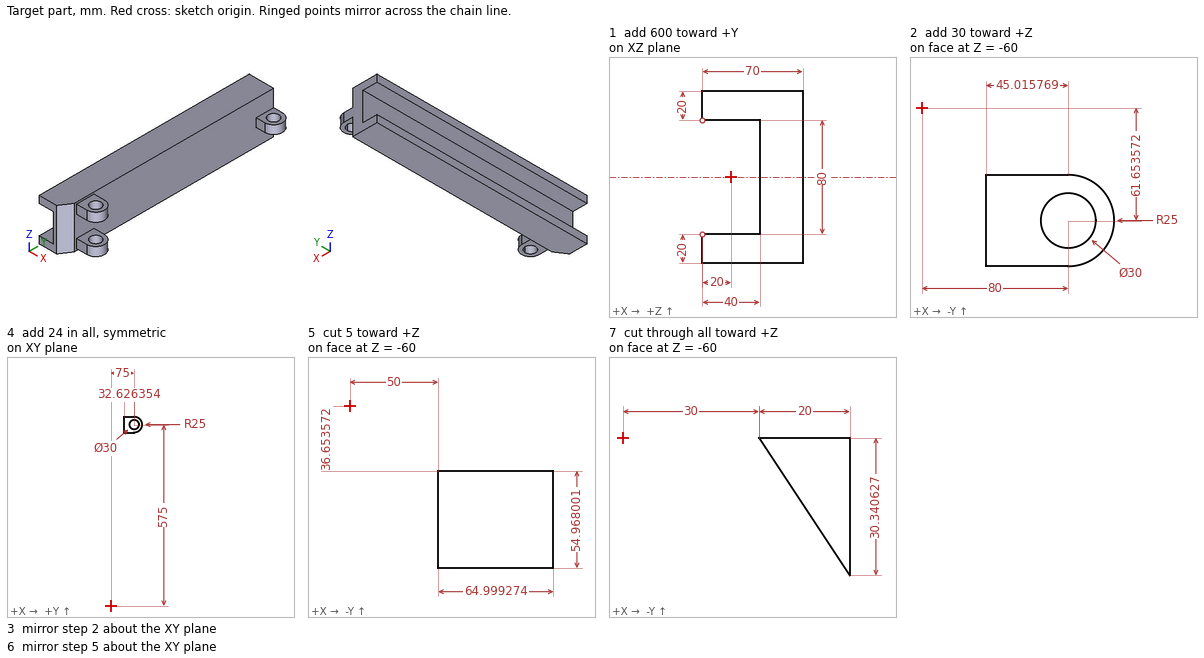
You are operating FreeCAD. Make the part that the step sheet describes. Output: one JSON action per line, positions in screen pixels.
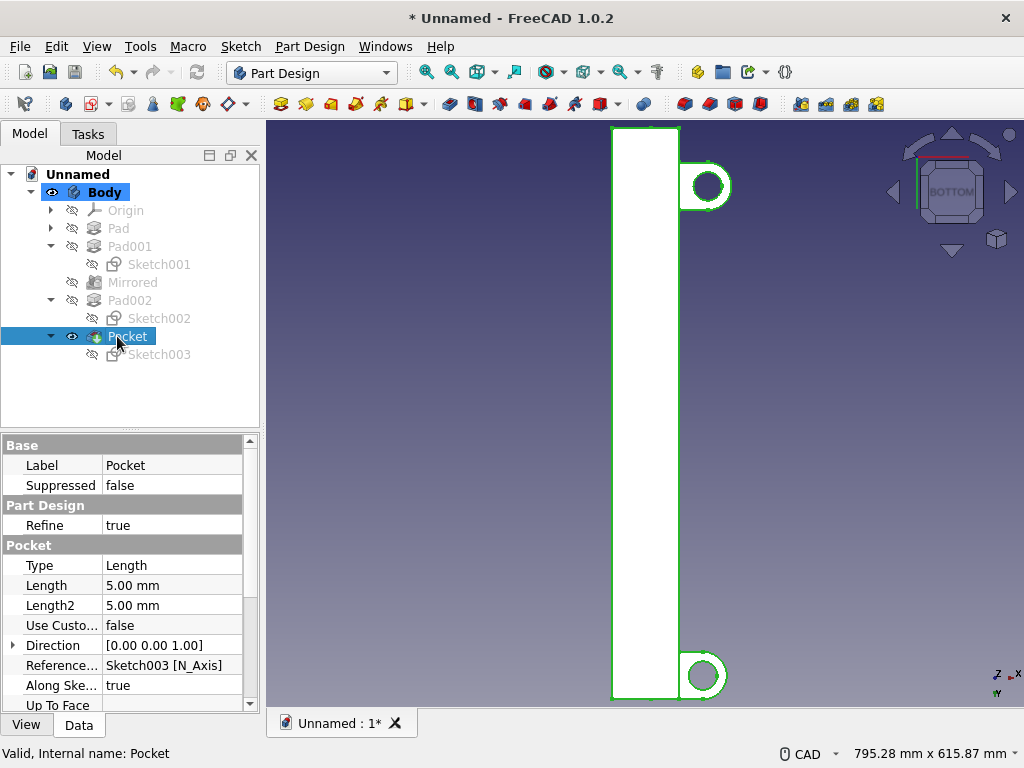
{"action": "left_click", "coordinate": [801, 104]}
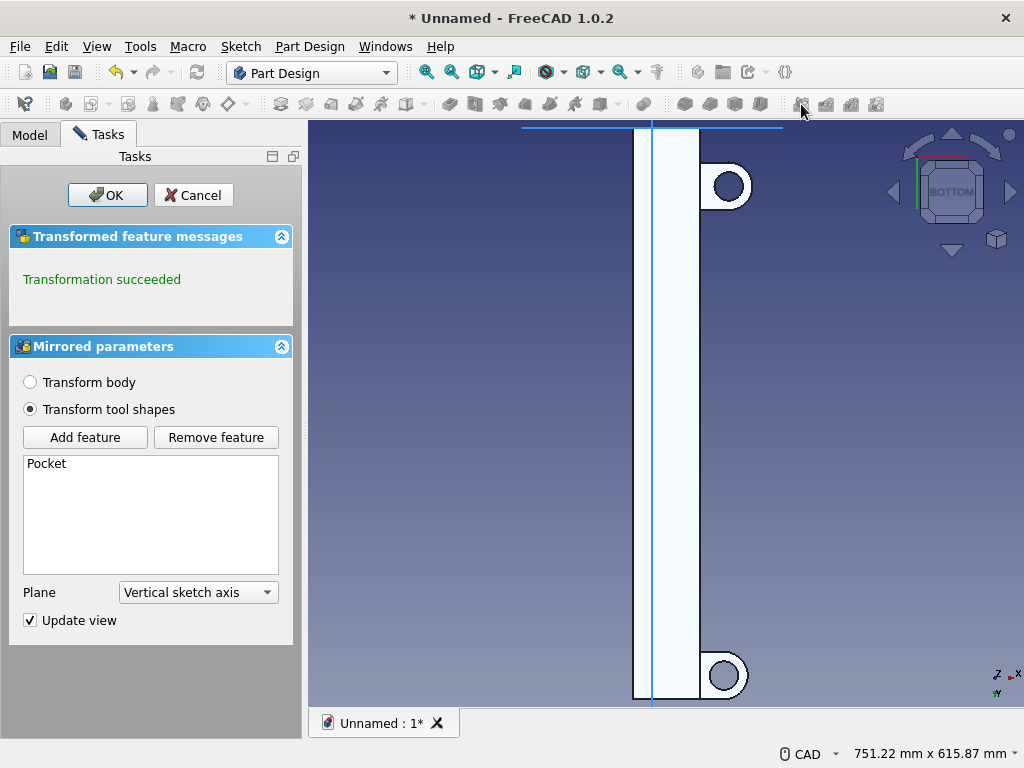
{"action": "left_click", "coordinate": [199, 592]}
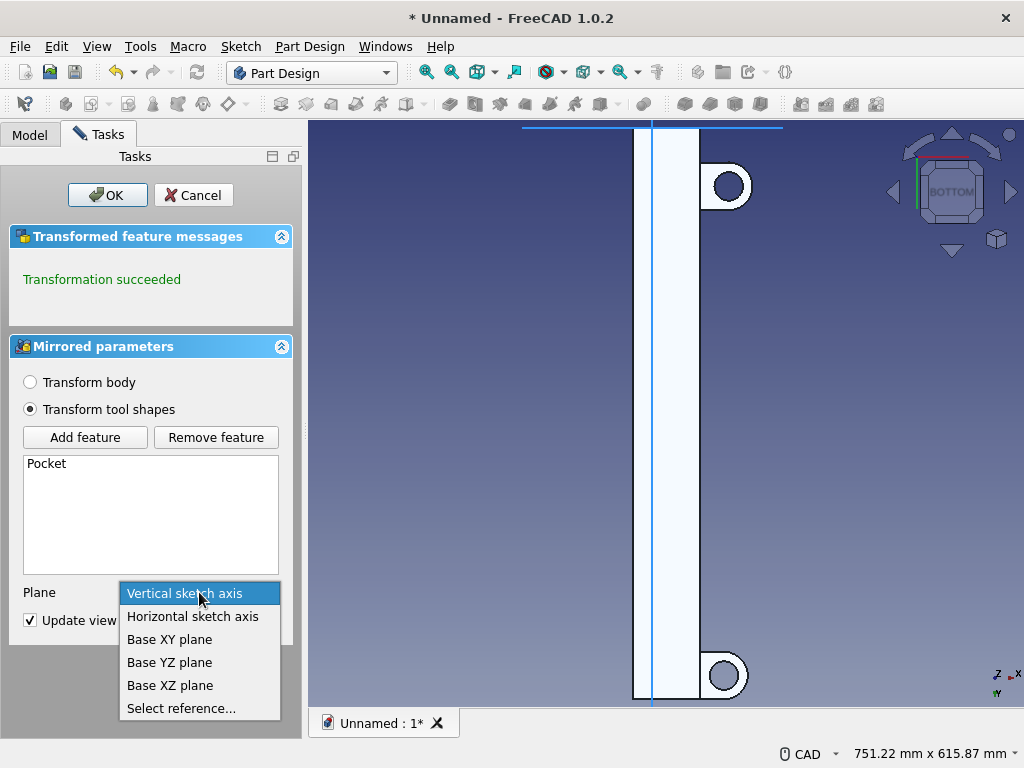
{"action": "left_click", "coordinate": [198, 640]}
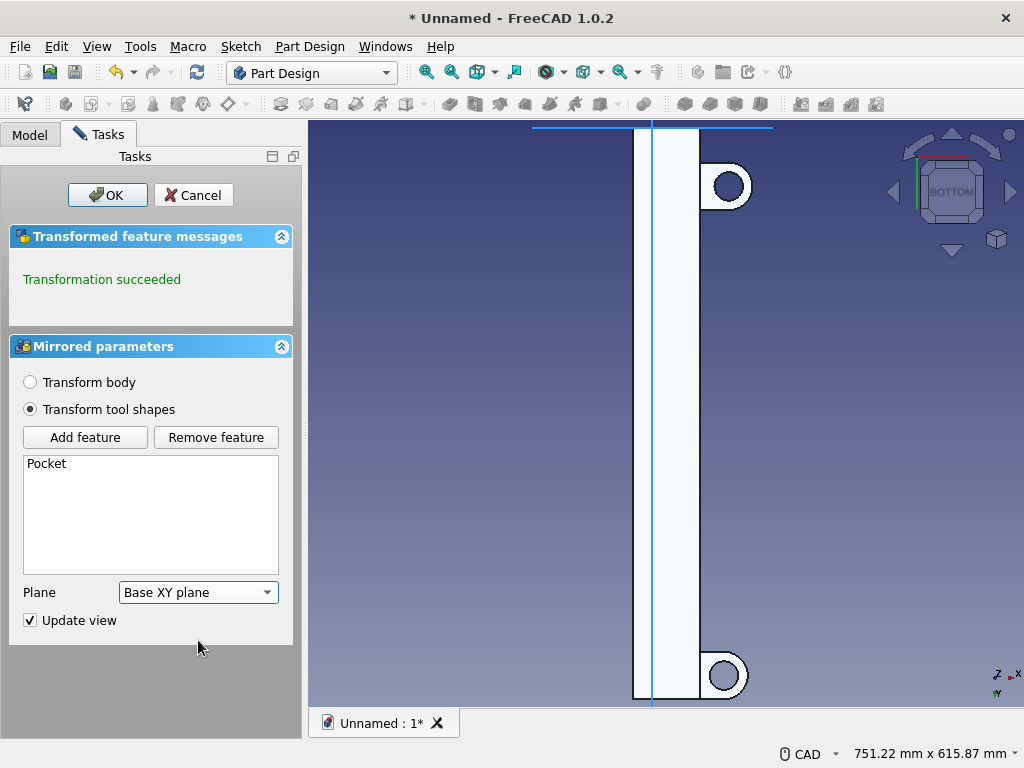
{"action": "left_click", "coordinate": [108, 195]}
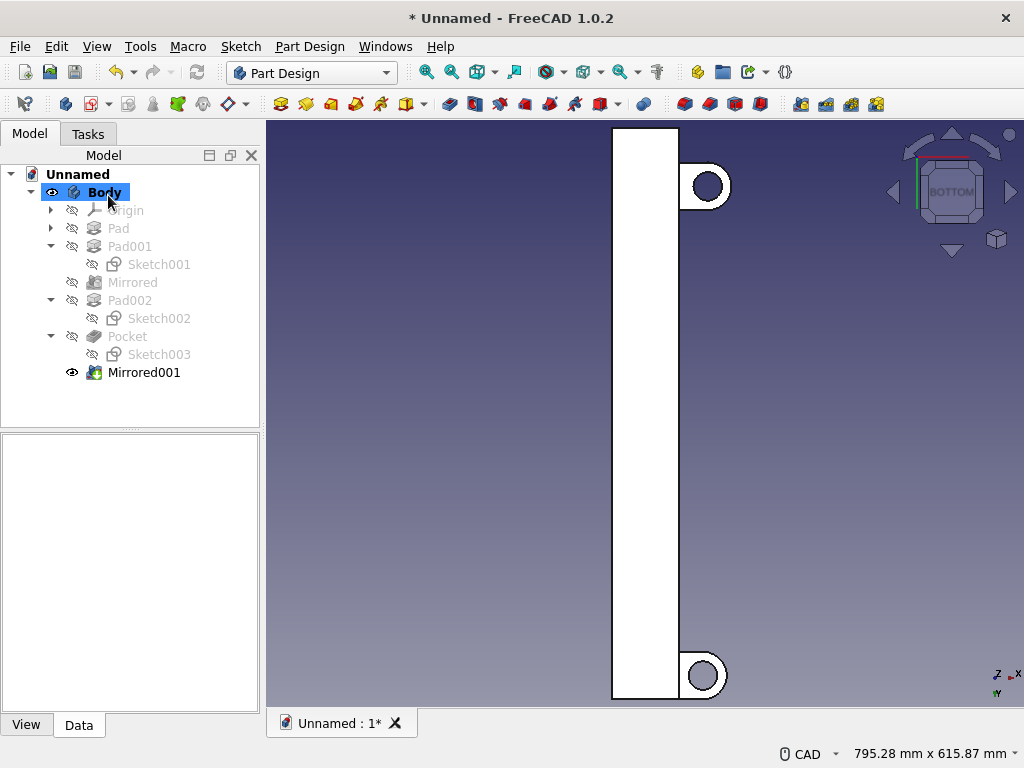
{"action": "left_click", "coordinate": [646, 658]}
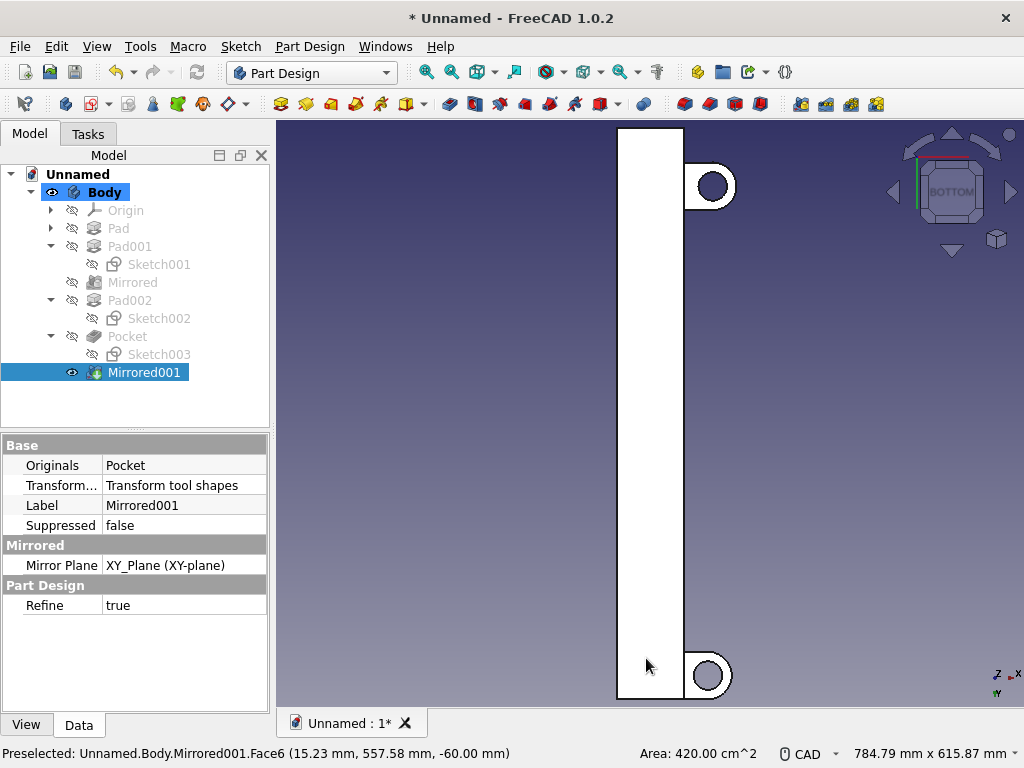
{"action": "left_click", "coordinate": [90, 104]}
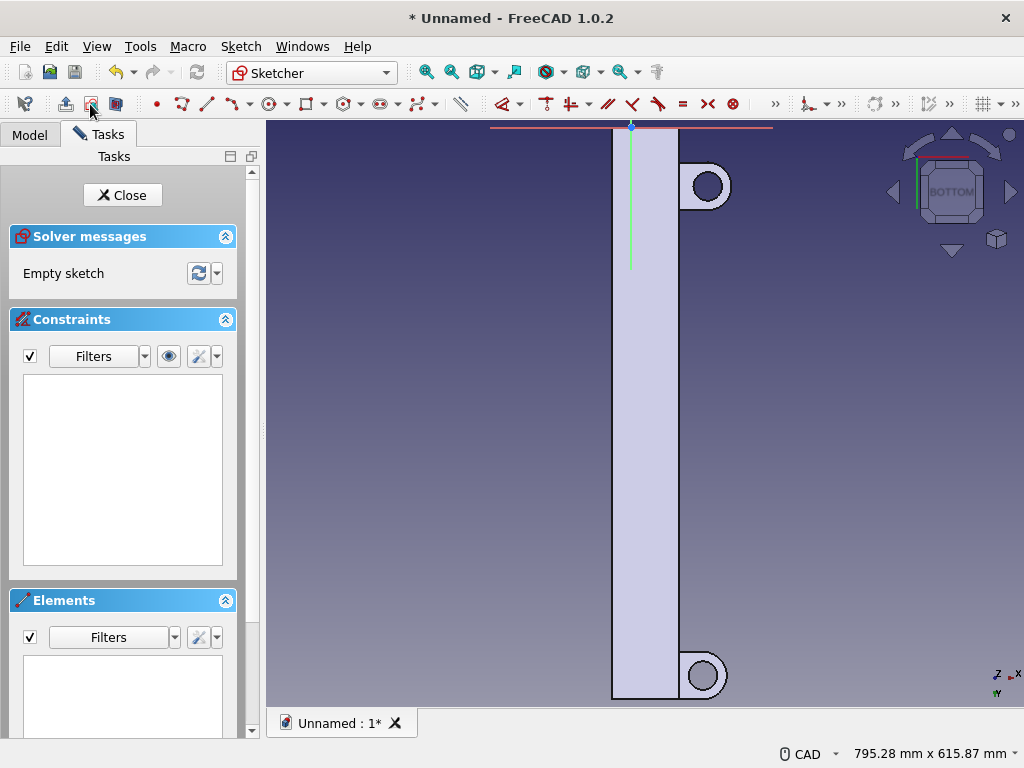
{"action": "scroll", "coordinate": [576, 414], "scroll_direction": "down", "scroll_amount": 5}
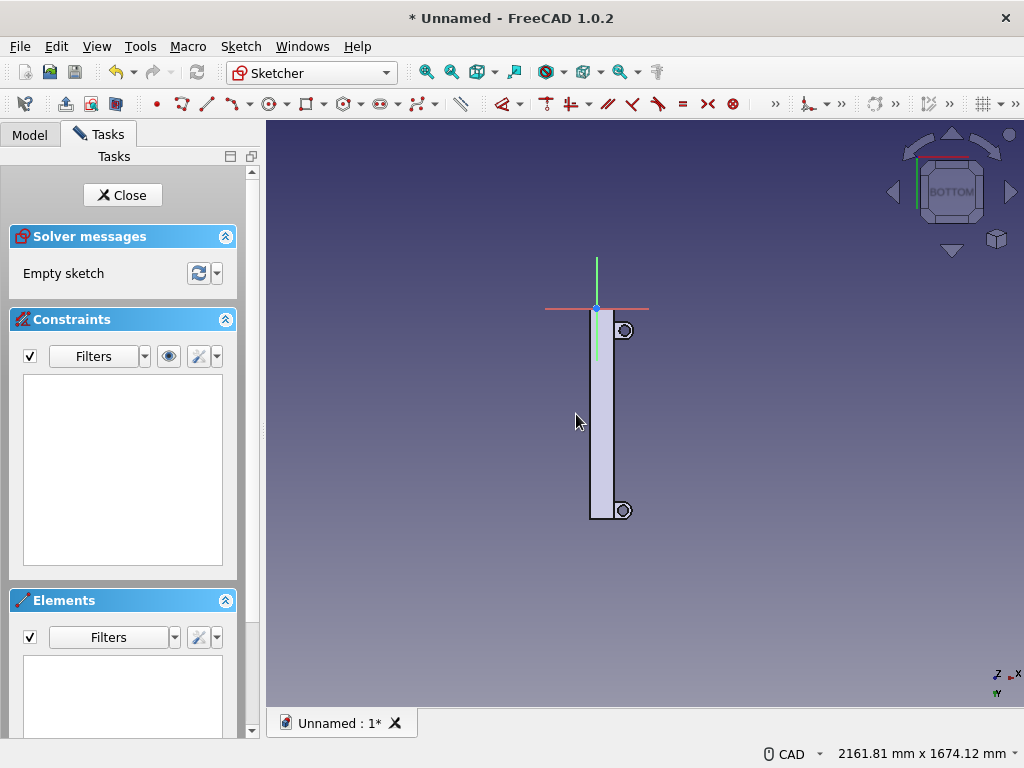
{"action": "scroll", "coordinate": [607, 309], "scroll_direction": "up", "scroll_amount": 15}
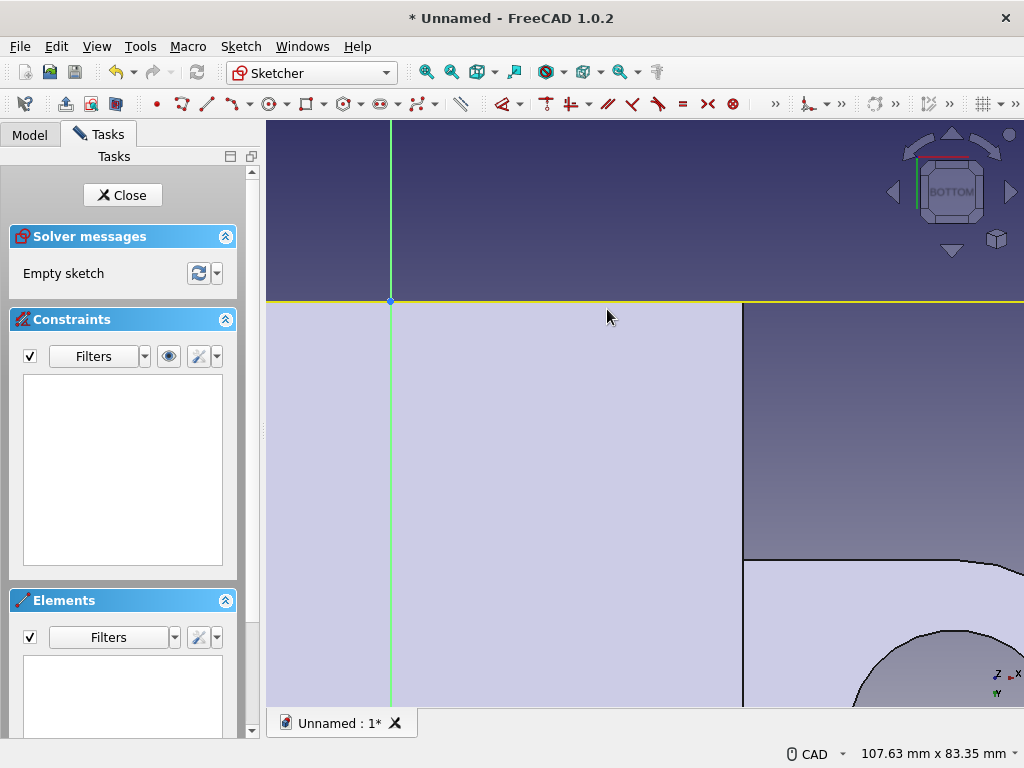
{"action": "left_click", "coordinate": [182, 104]}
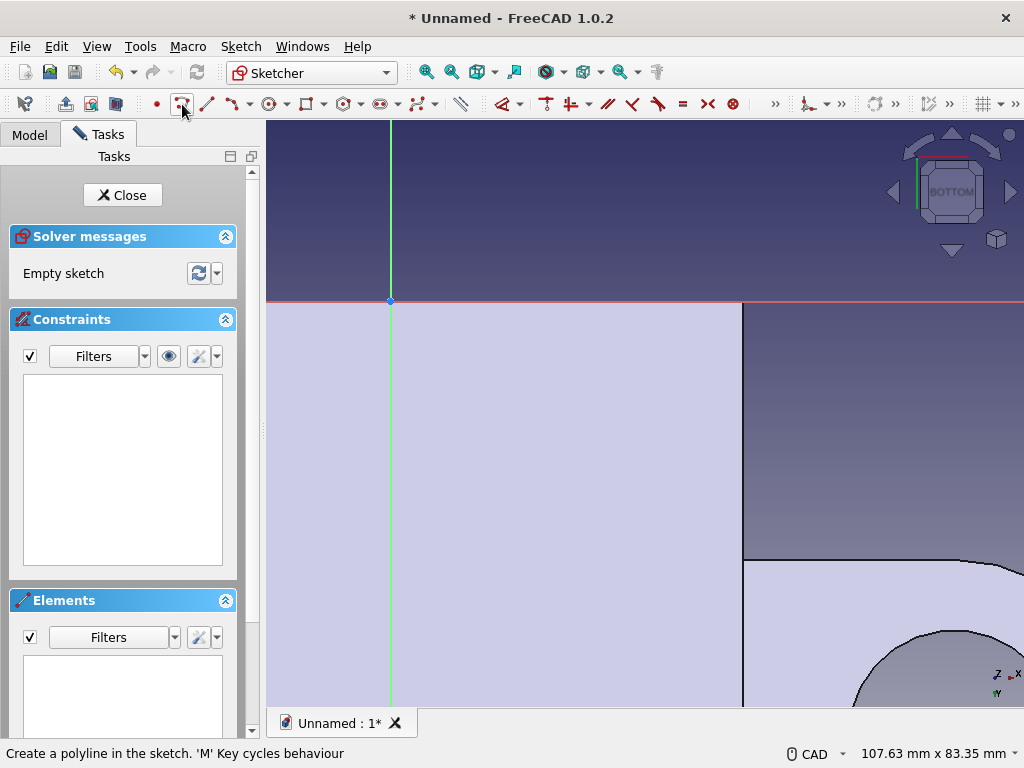
{"action": "left_click", "coordinate": [602, 302]}
{"action": "left_click", "coordinate": [743, 515]}
{"action": "left_click", "coordinate": [743, 311]}
{"action": "left_click", "coordinate": [602, 302]}
{"action": "key", "text": "Escape"}
{"action": "key", "text": "Escape"}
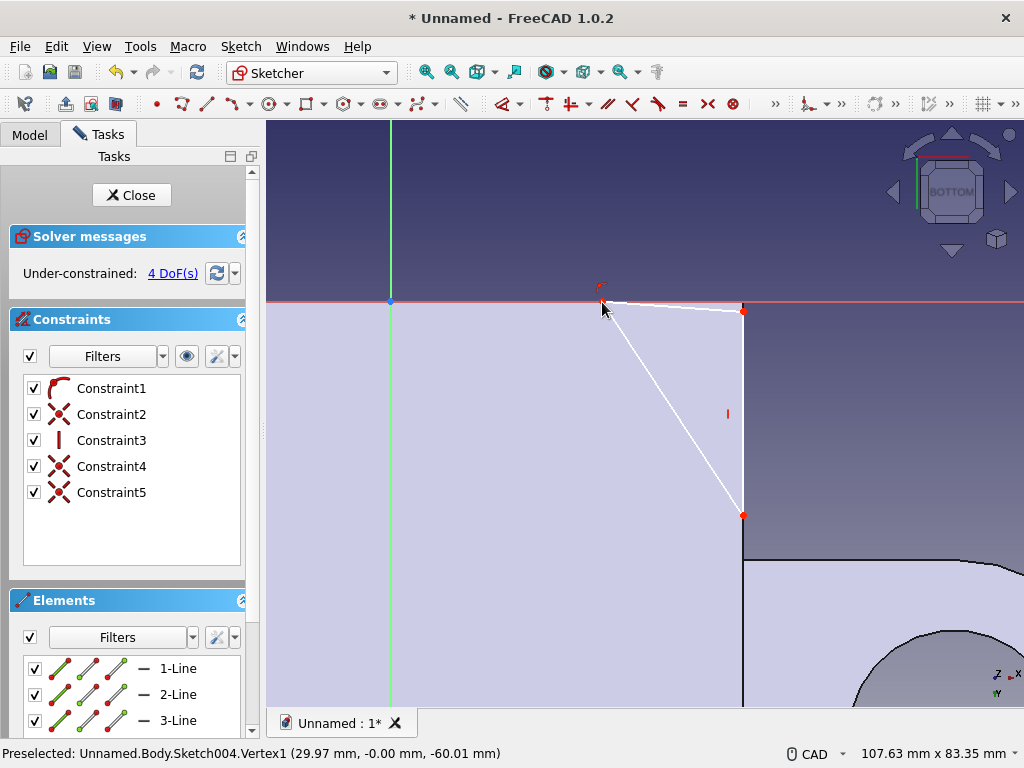
{"action": "left_click", "coordinate": [644, 305]}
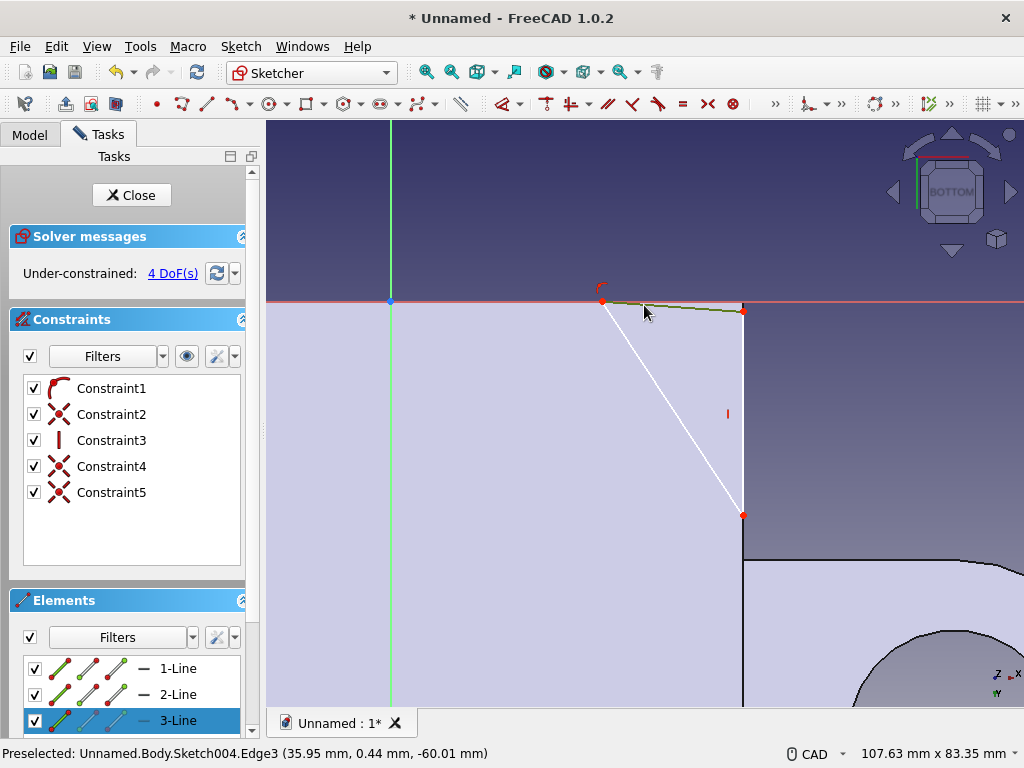
{"action": "left_click", "coordinate": [588, 104]}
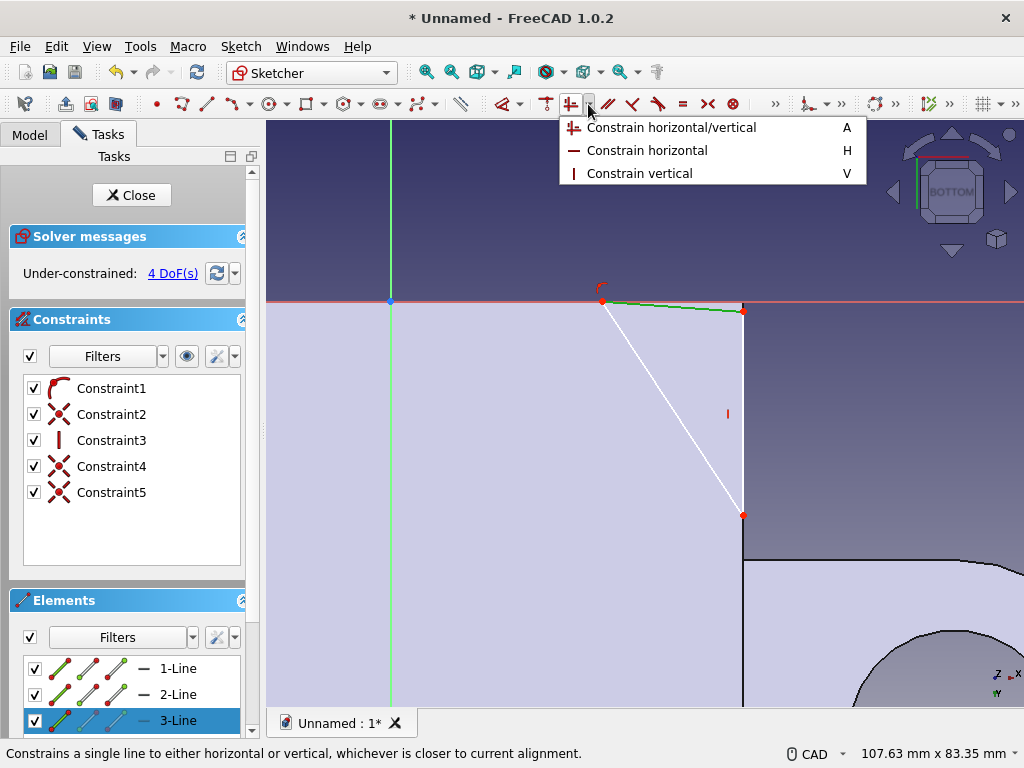
{"action": "left_click", "coordinate": [713, 150]}